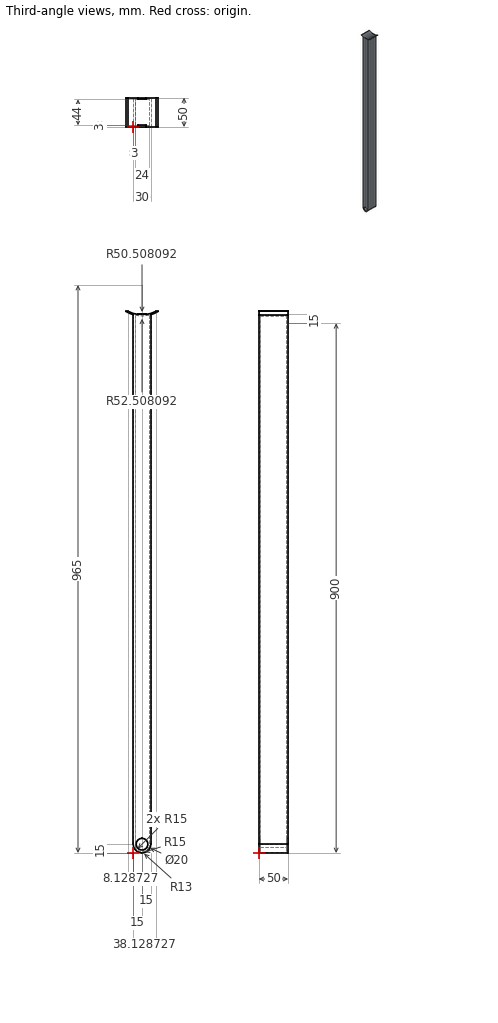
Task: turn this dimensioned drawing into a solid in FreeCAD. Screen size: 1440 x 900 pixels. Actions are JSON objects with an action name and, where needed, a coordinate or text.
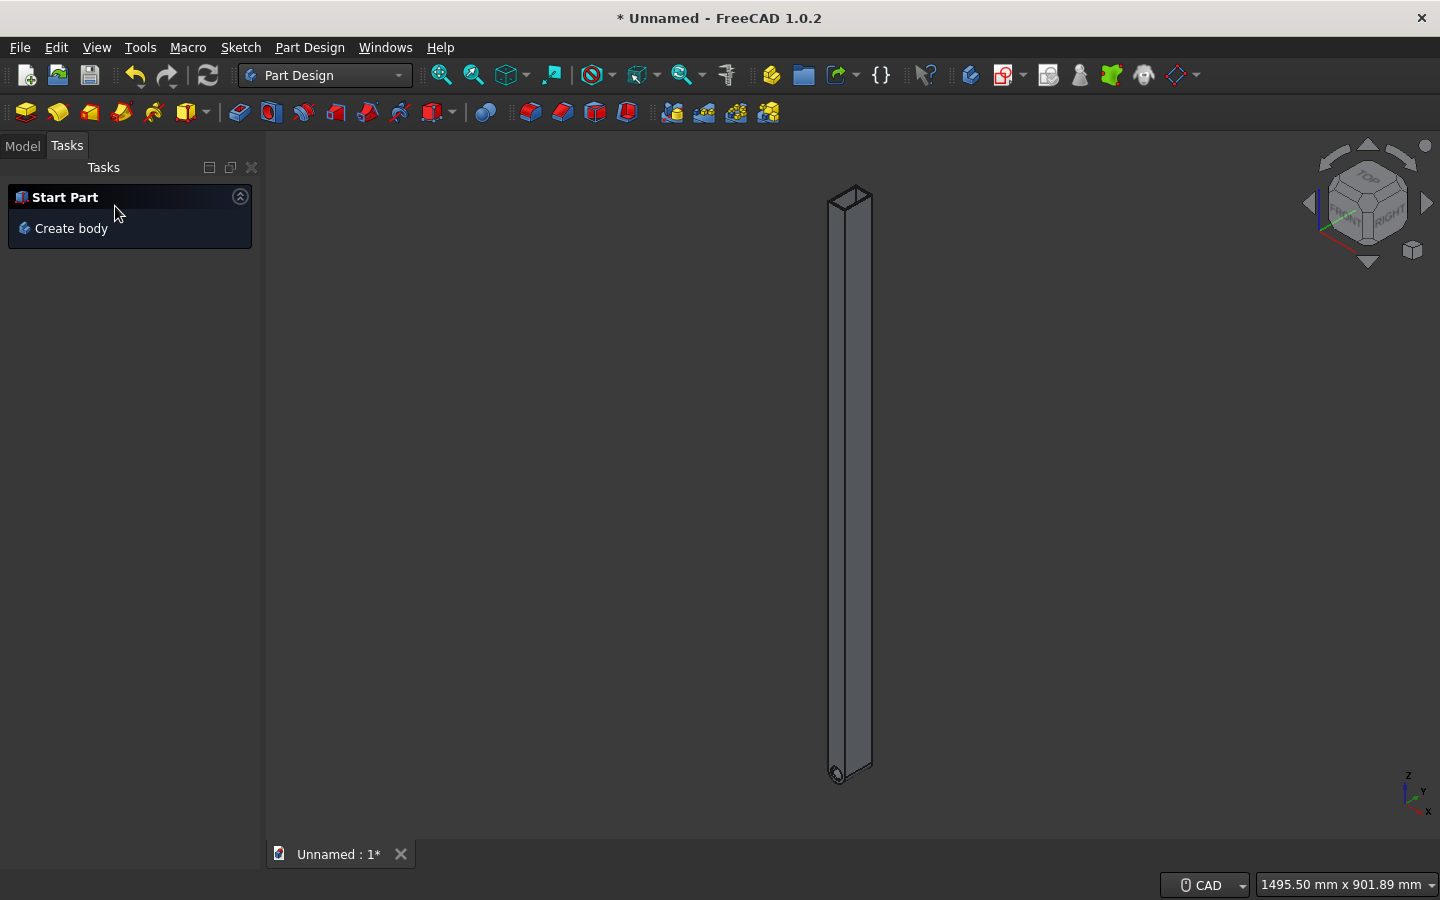
{"action": "scroll", "coordinate": [869, 194], "scroll_direction": "up", "scroll_amount": 15}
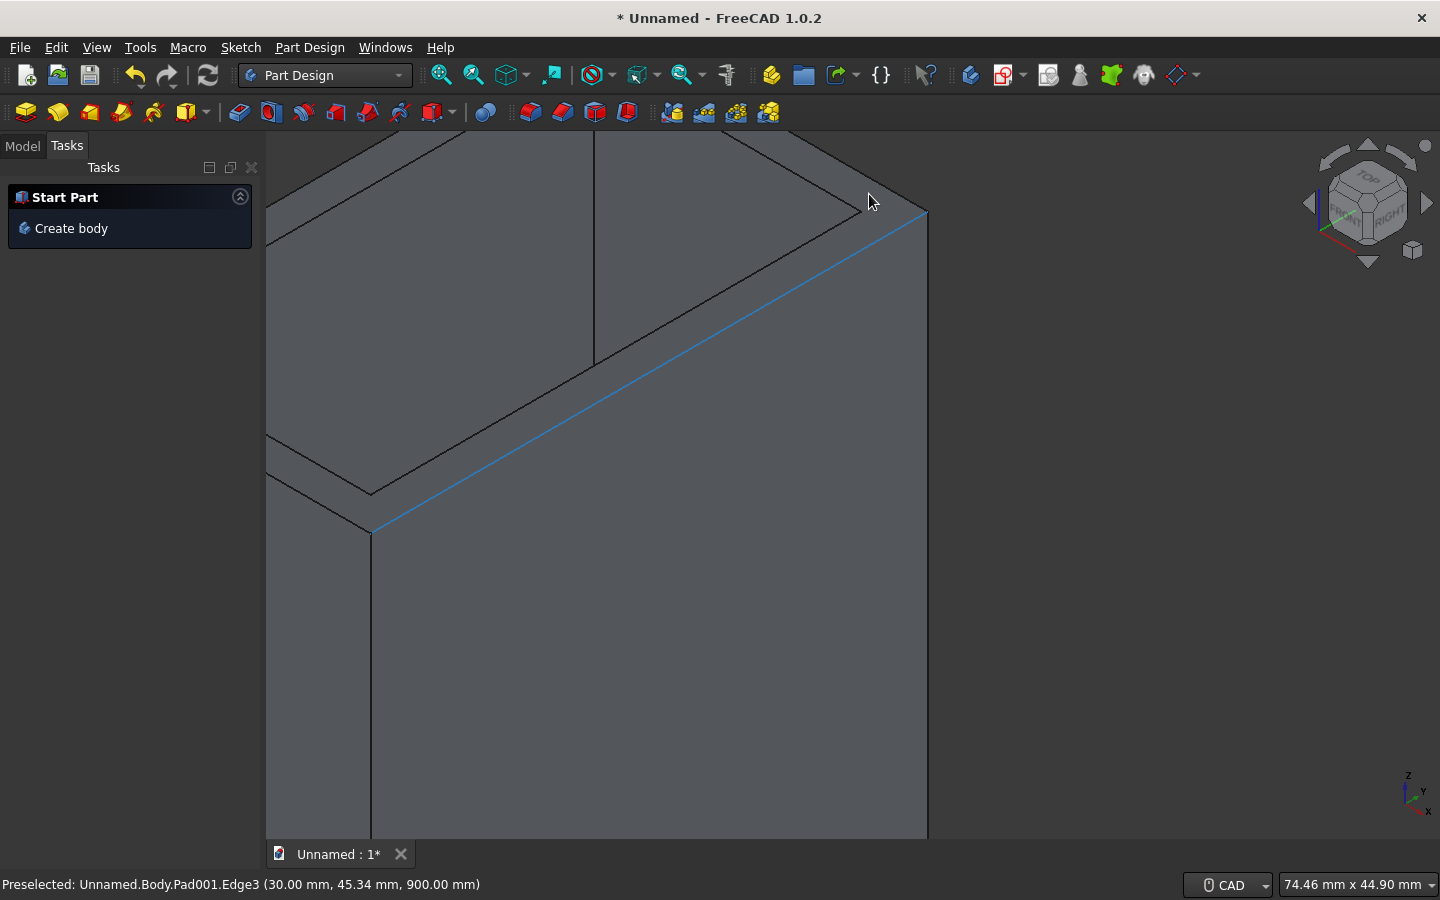
{"action": "left_click", "coordinate": [864, 220]}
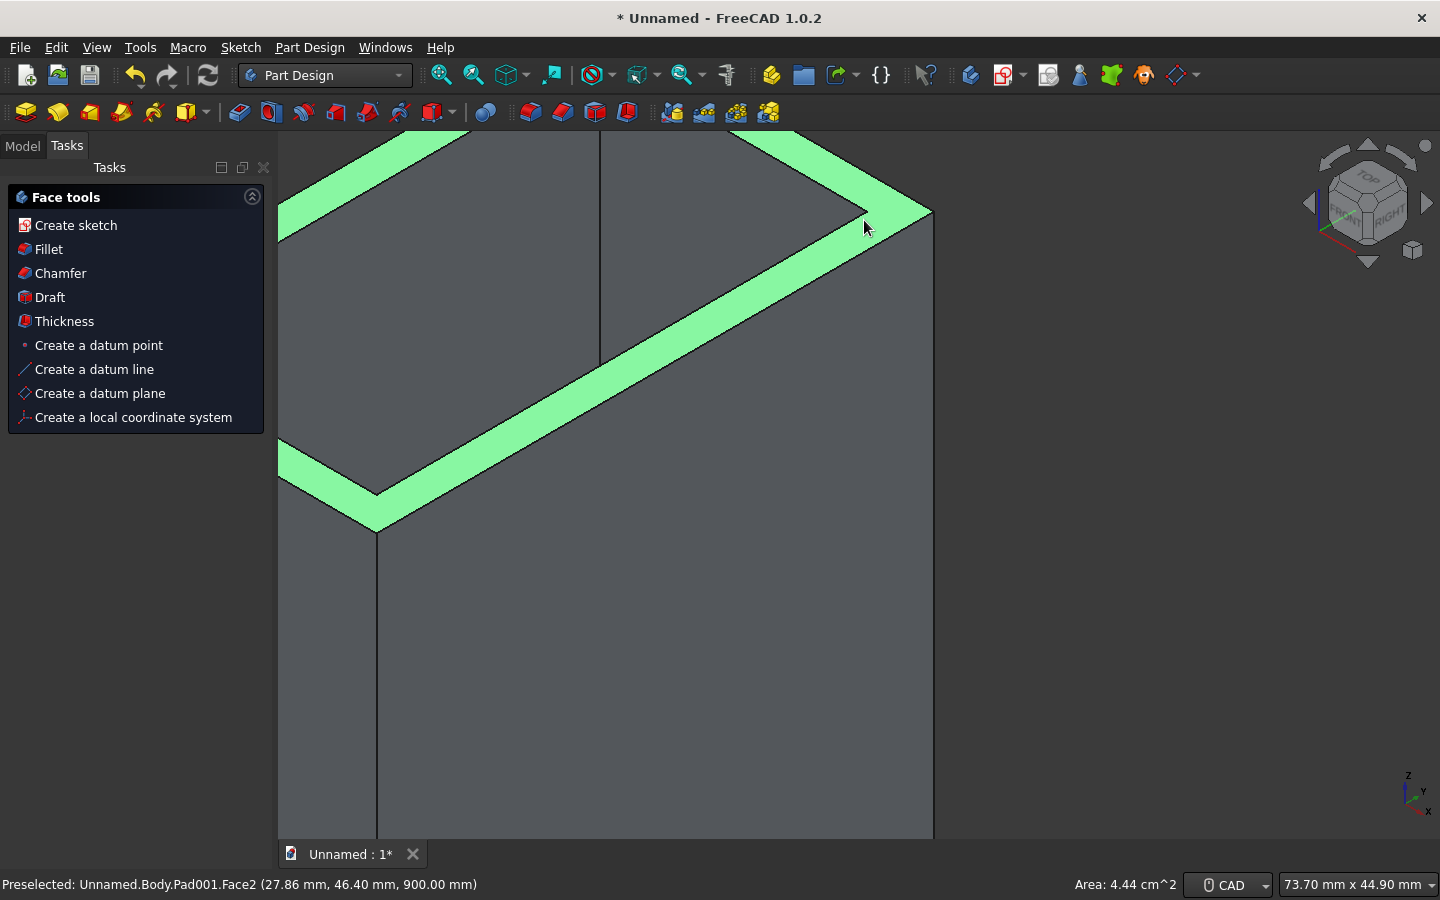
{"action": "left_click", "coordinate": [1004, 76]}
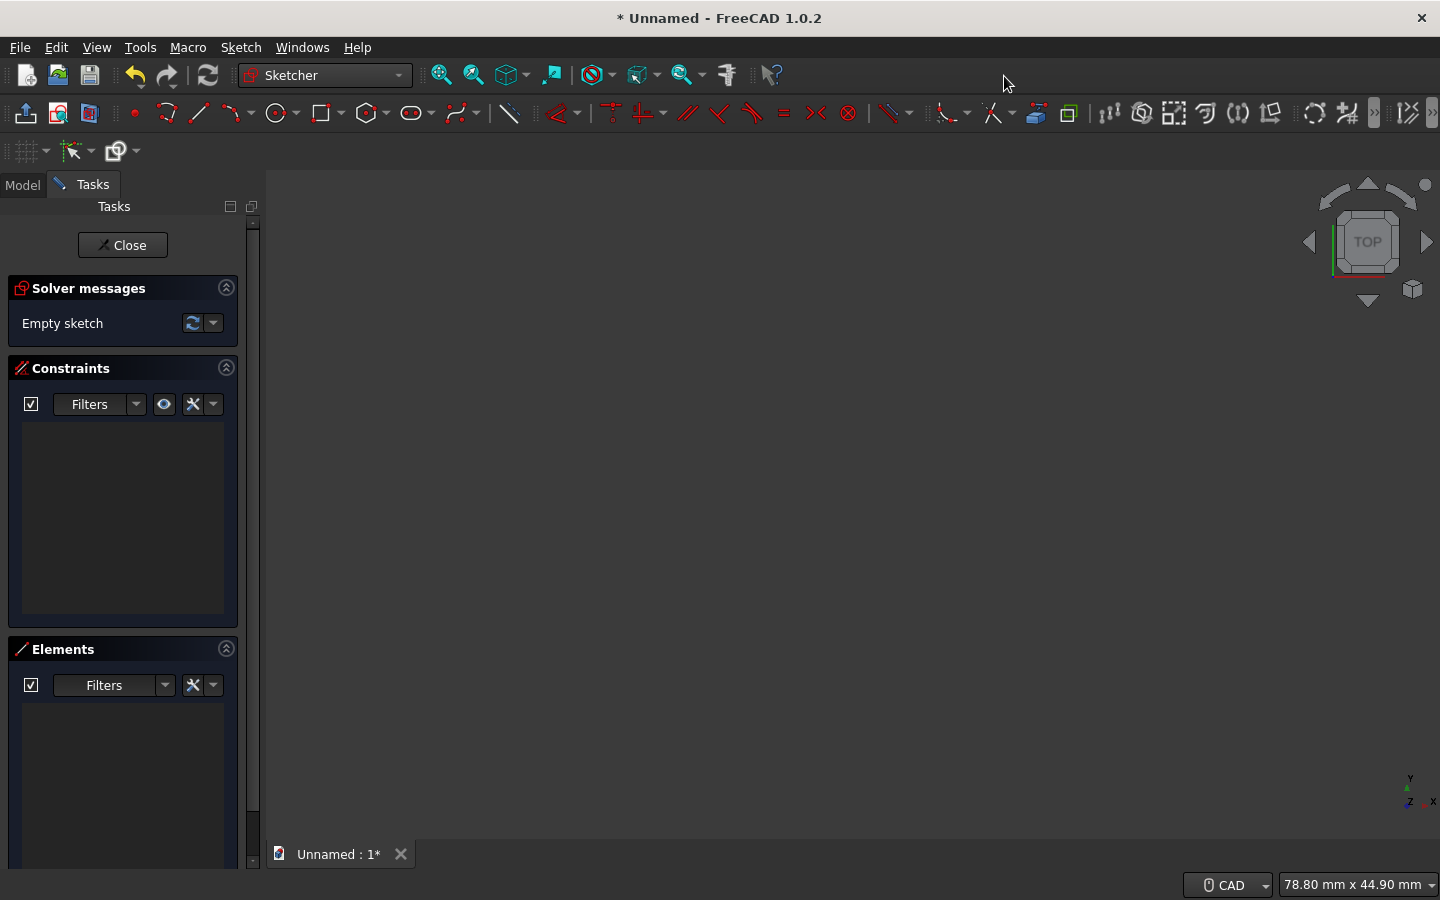
{"action": "scroll", "coordinate": [784, 504], "scroll_direction": "down", "scroll_amount": 5}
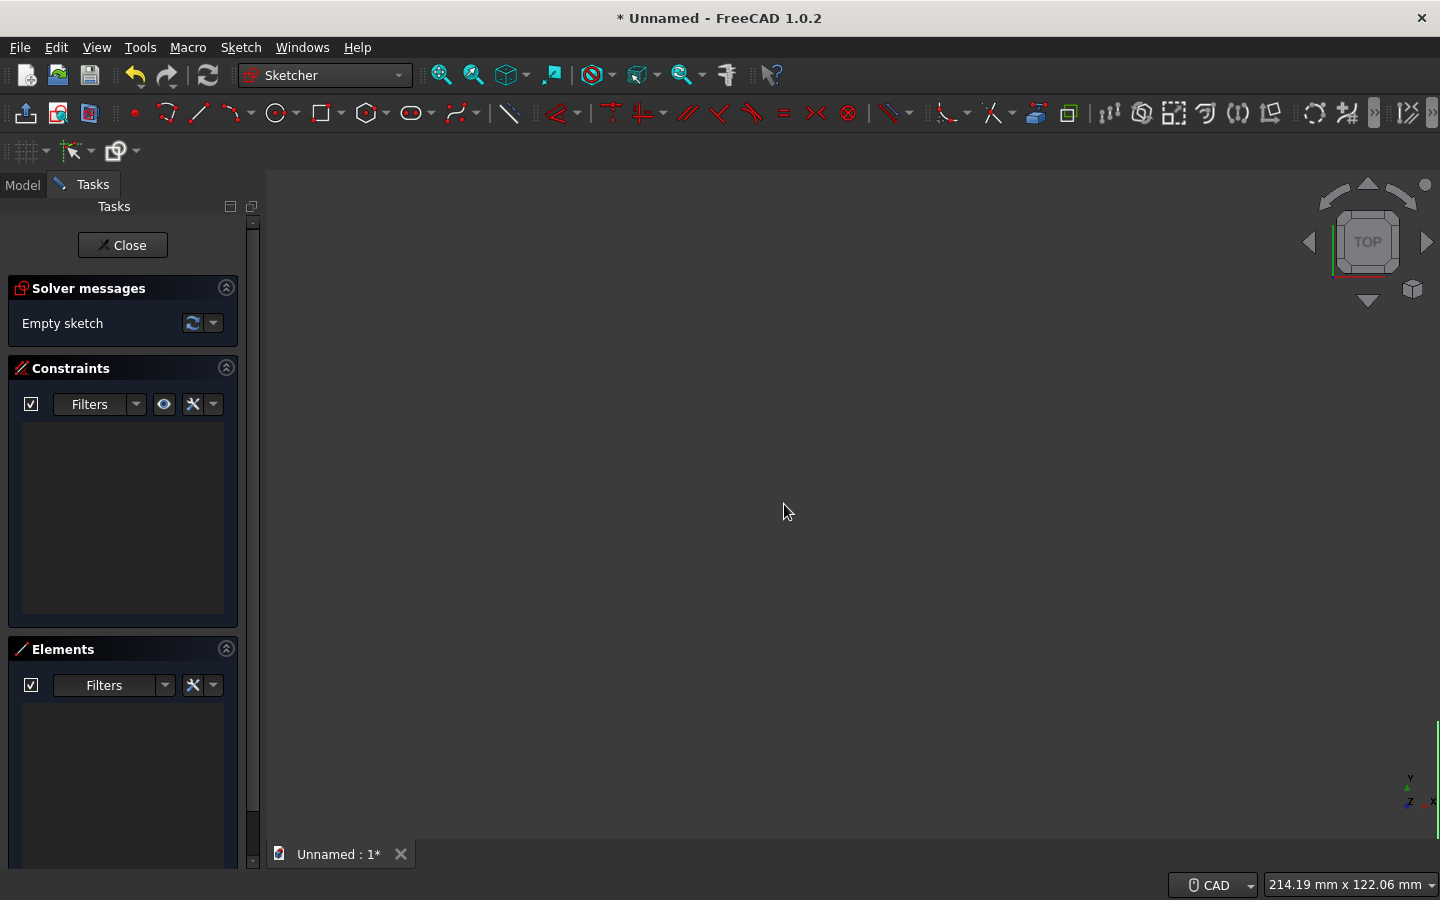
{"action": "scroll", "coordinate": [784, 504], "scroll_direction": "down", "scroll_amount": 5}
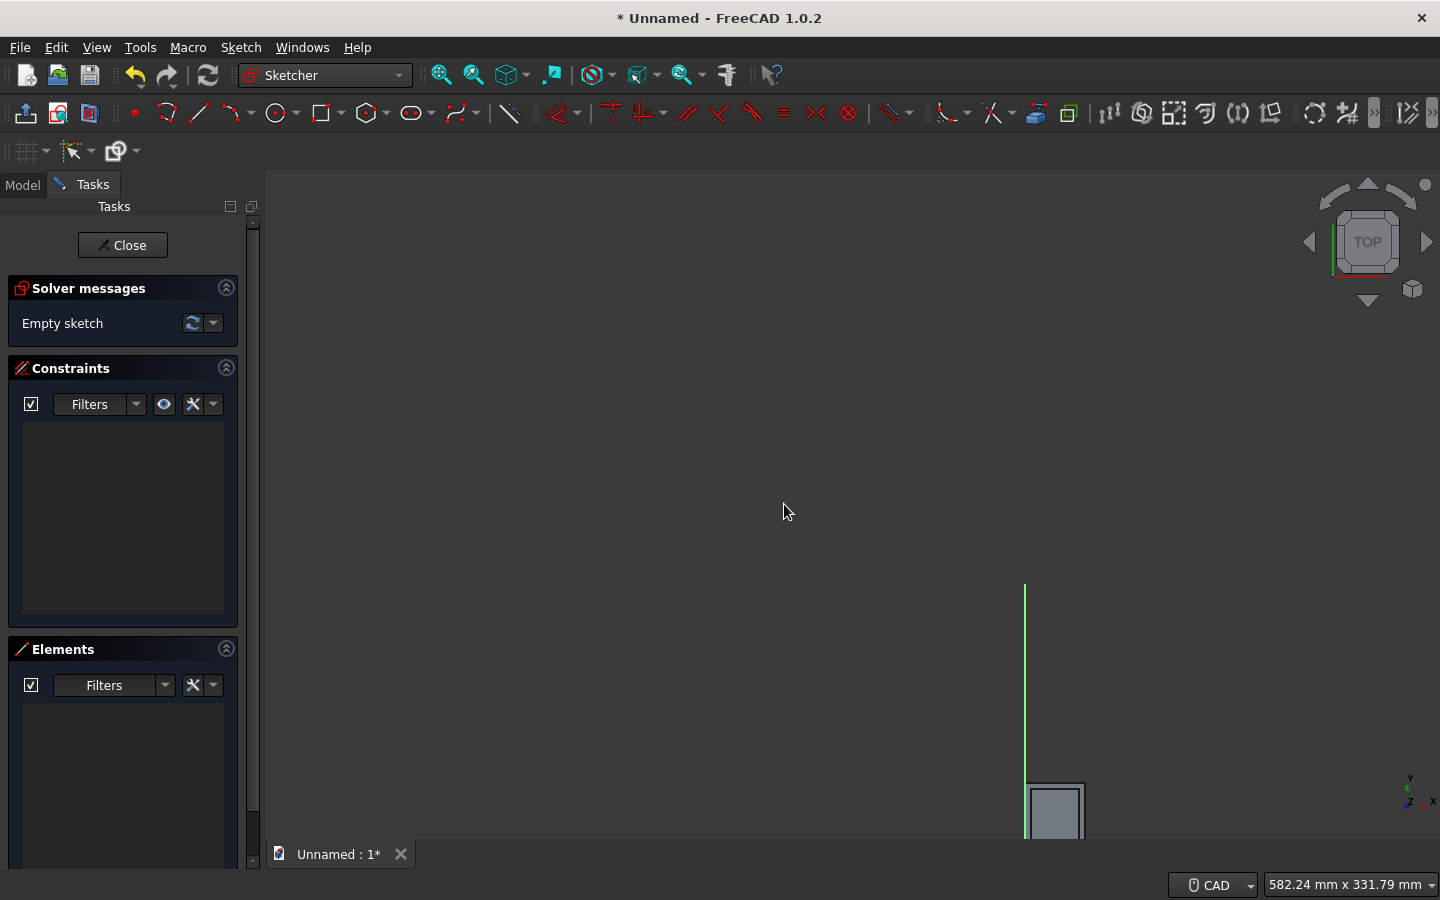
{"action": "scroll", "coordinate": [784, 504], "scroll_direction": "down", "scroll_amount": 5}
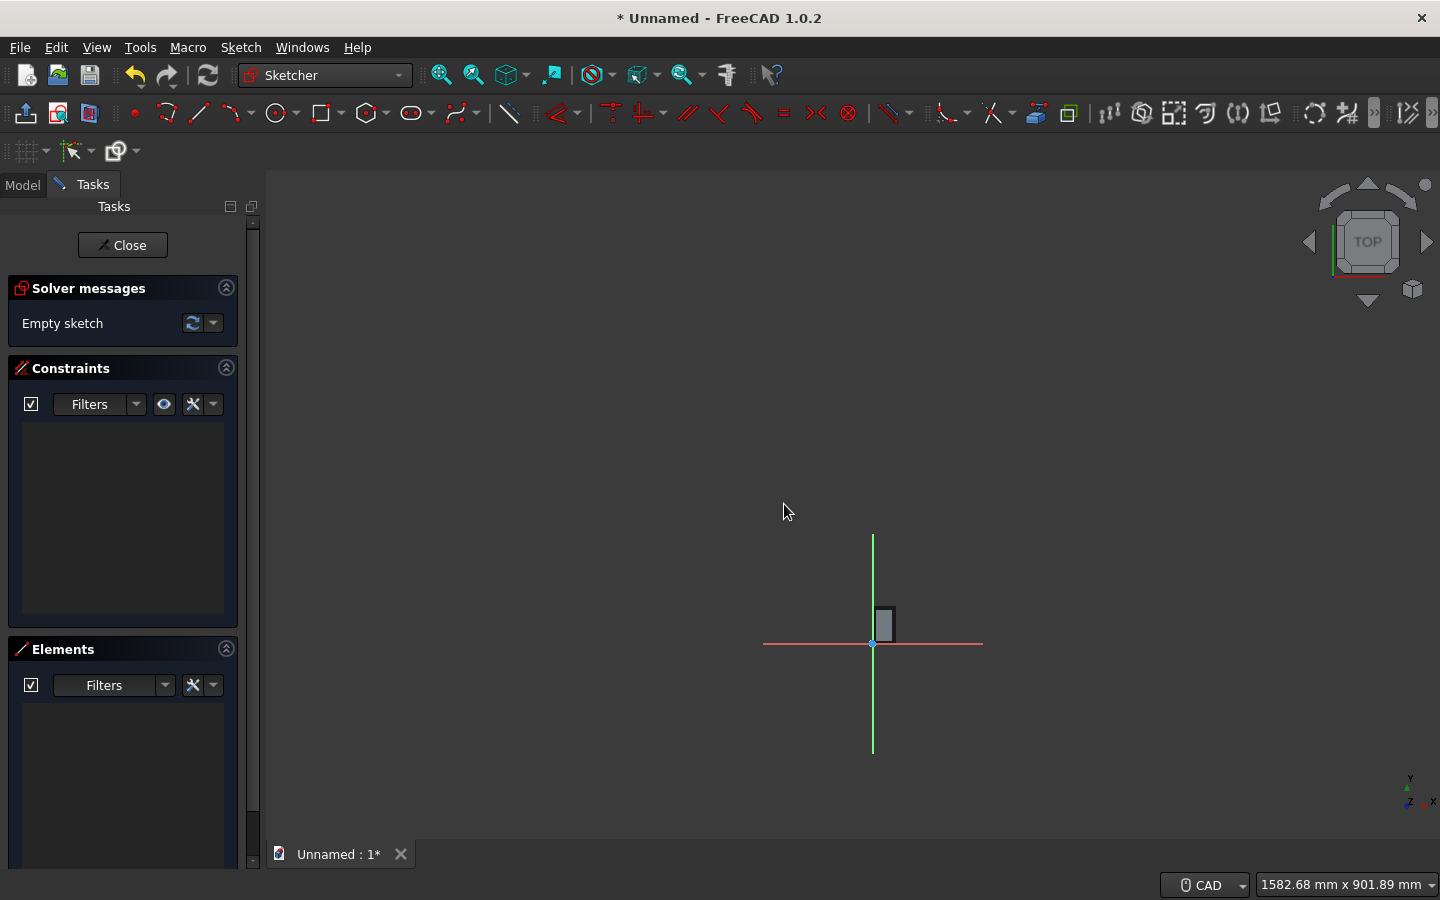
{"action": "scroll", "coordinate": [894, 637], "scroll_direction": "up", "scroll_amount": 12}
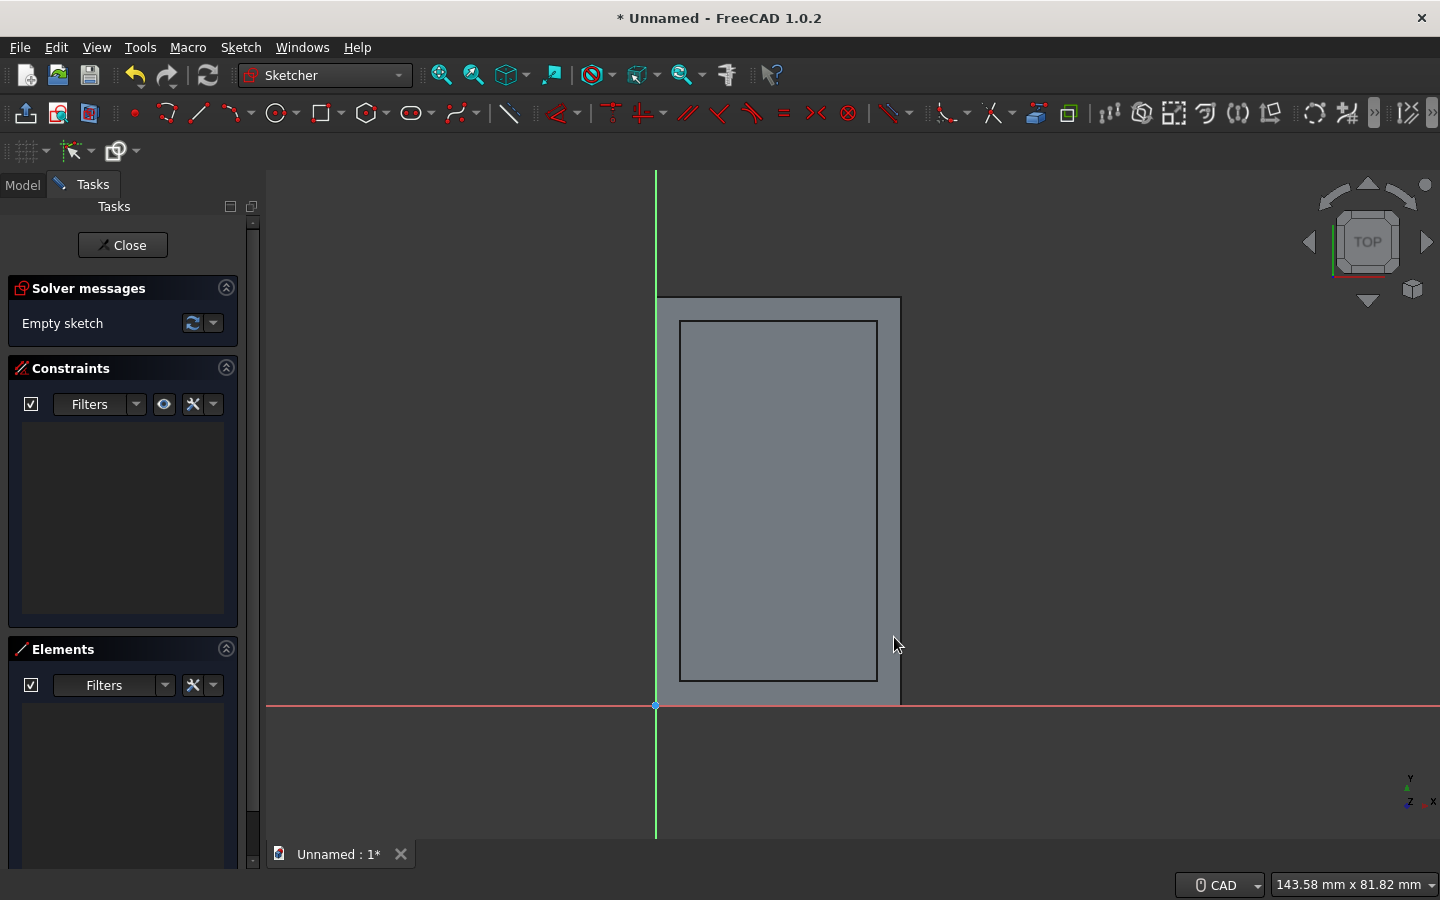
{"action": "left_click", "coordinate": [322, 114]}